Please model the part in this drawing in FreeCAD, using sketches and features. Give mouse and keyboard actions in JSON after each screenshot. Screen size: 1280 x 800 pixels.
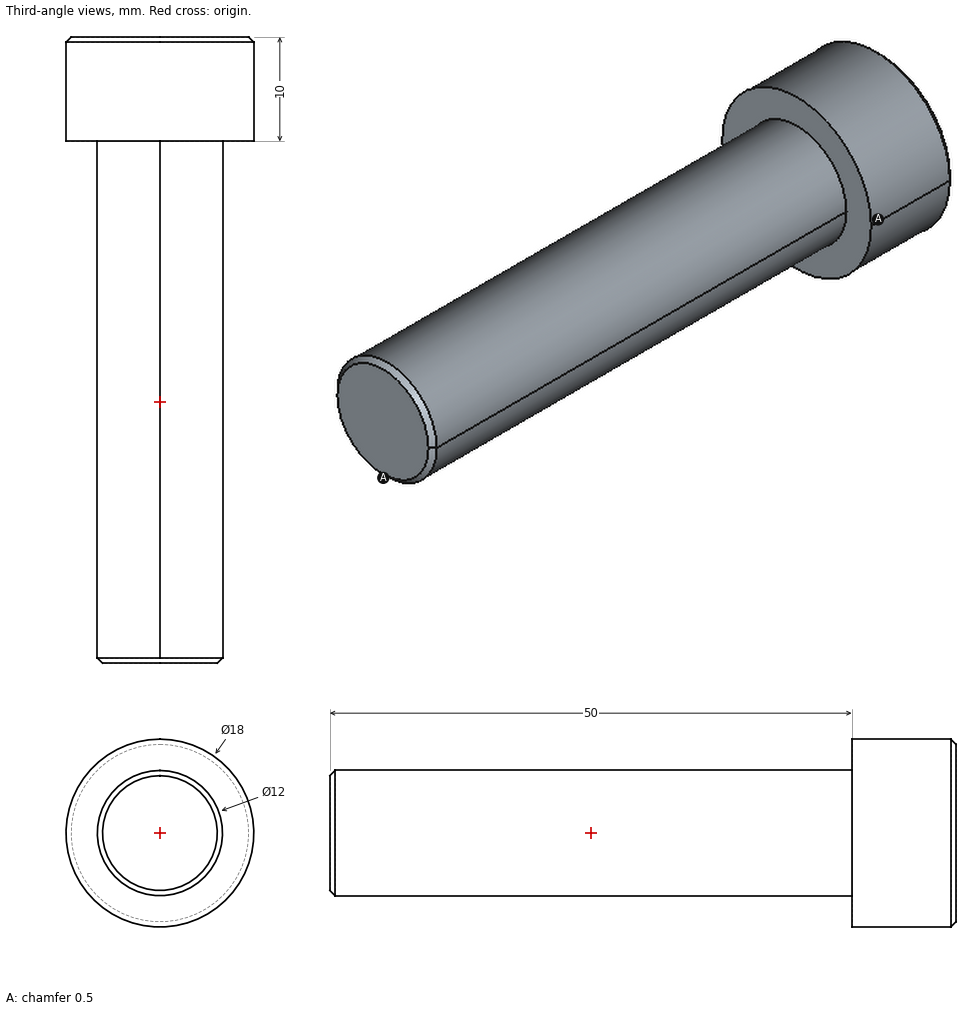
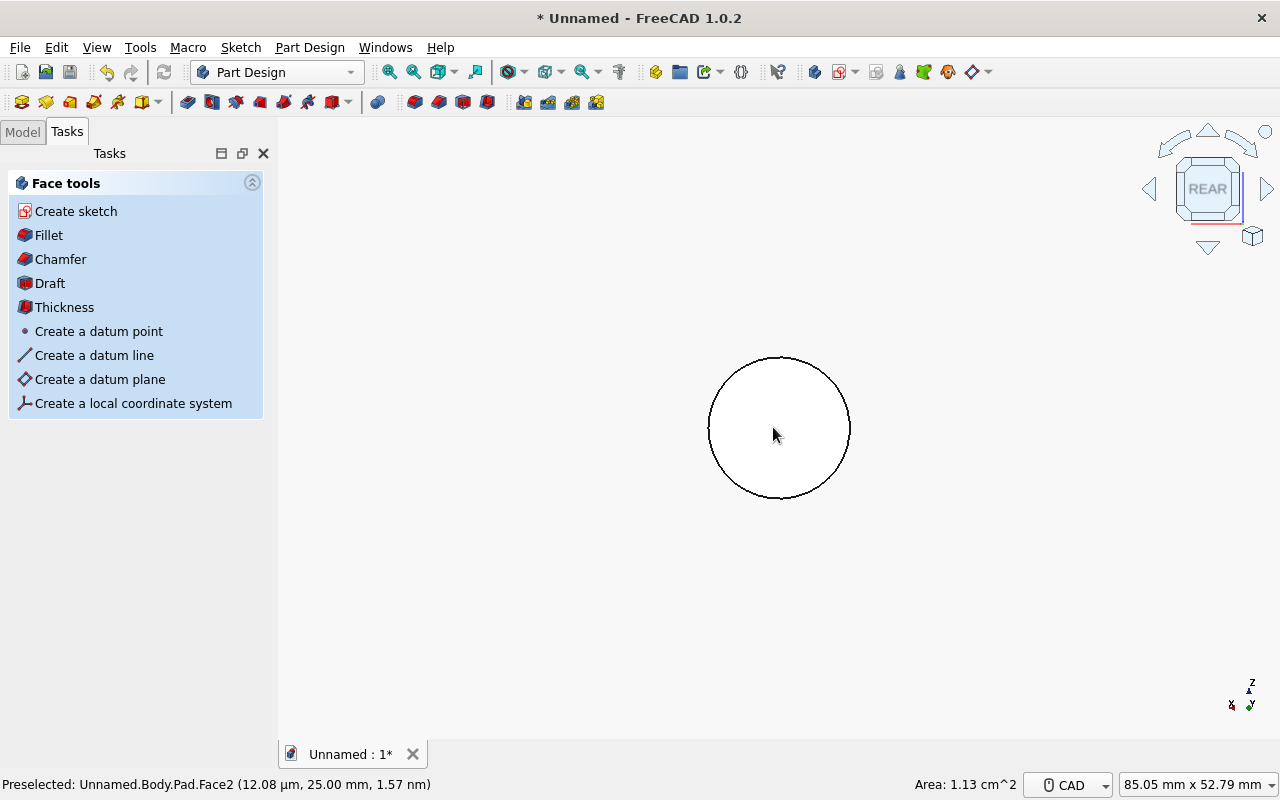
{"action": "left_click", "coordinate": [840, 72]}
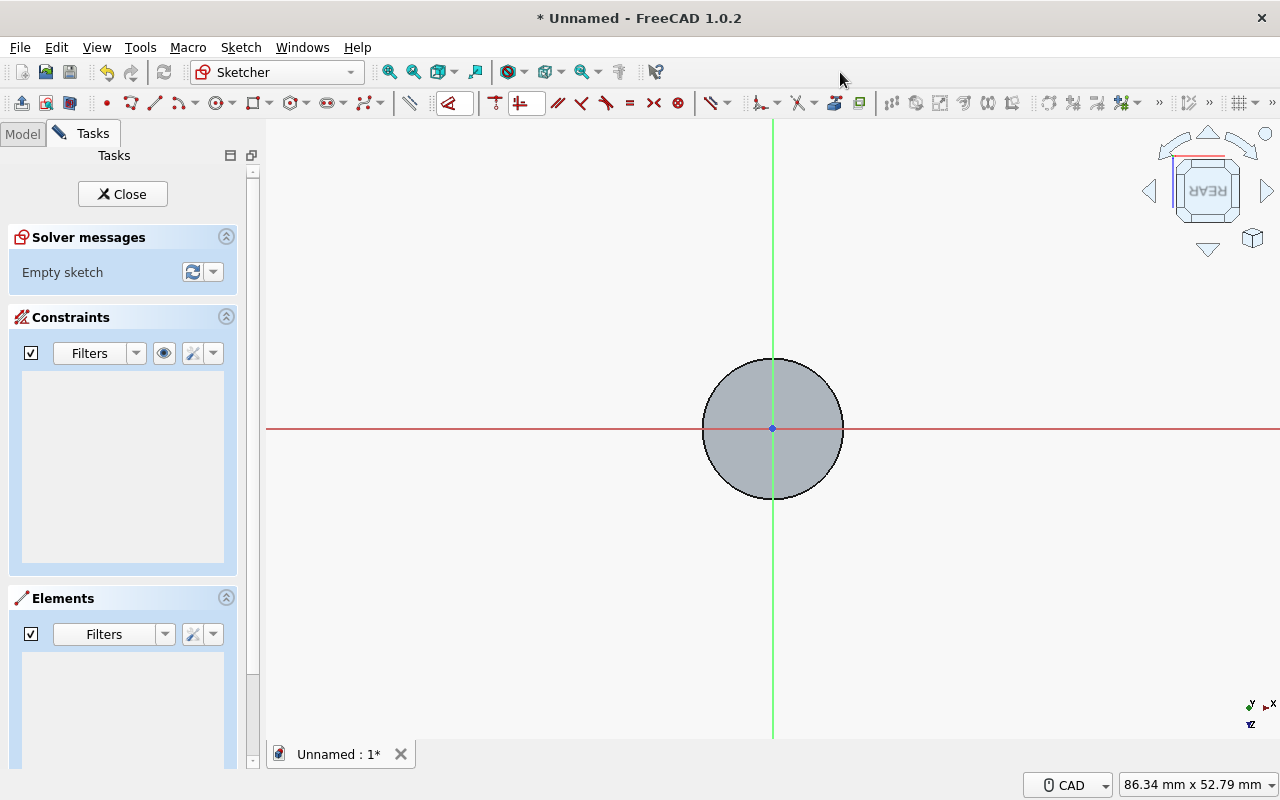
{"action": "scroll", "coordinate": [856, 429], "scroll_direction": "up", "scroll_amount": 3}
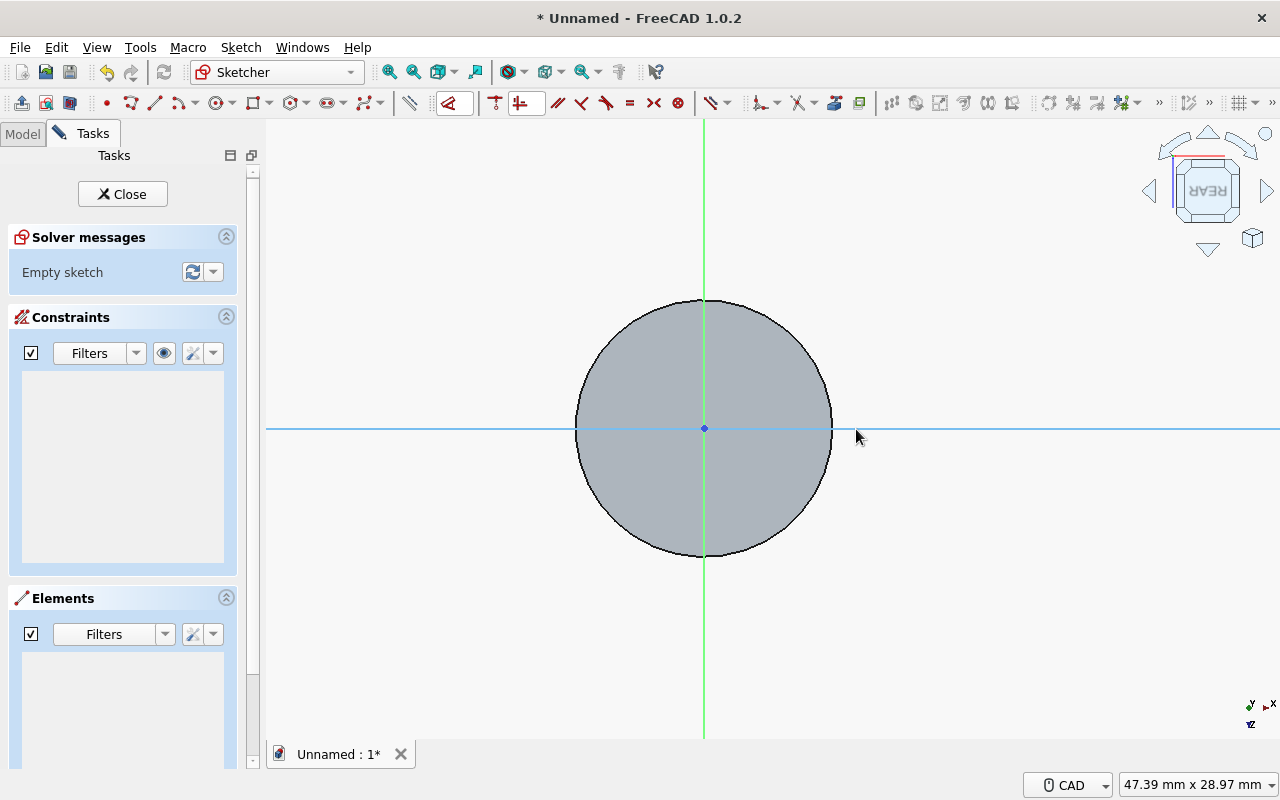
{"action": "left_click", "coordinate": [216, 104]}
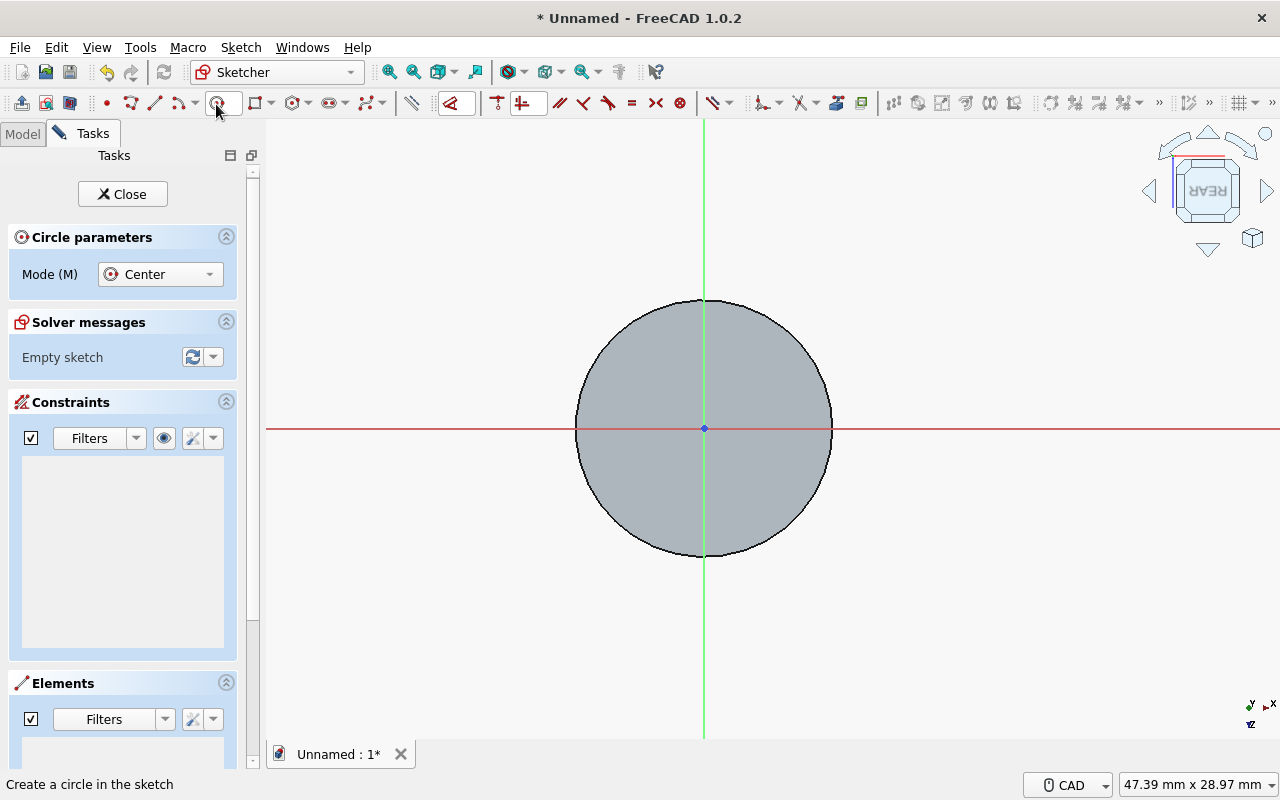
{"action": "left_click", "coordinate": [704, 429]}
{"action": "left_click", "coordinate": [840, 292]}
{"action": "key", "text": "Escape"}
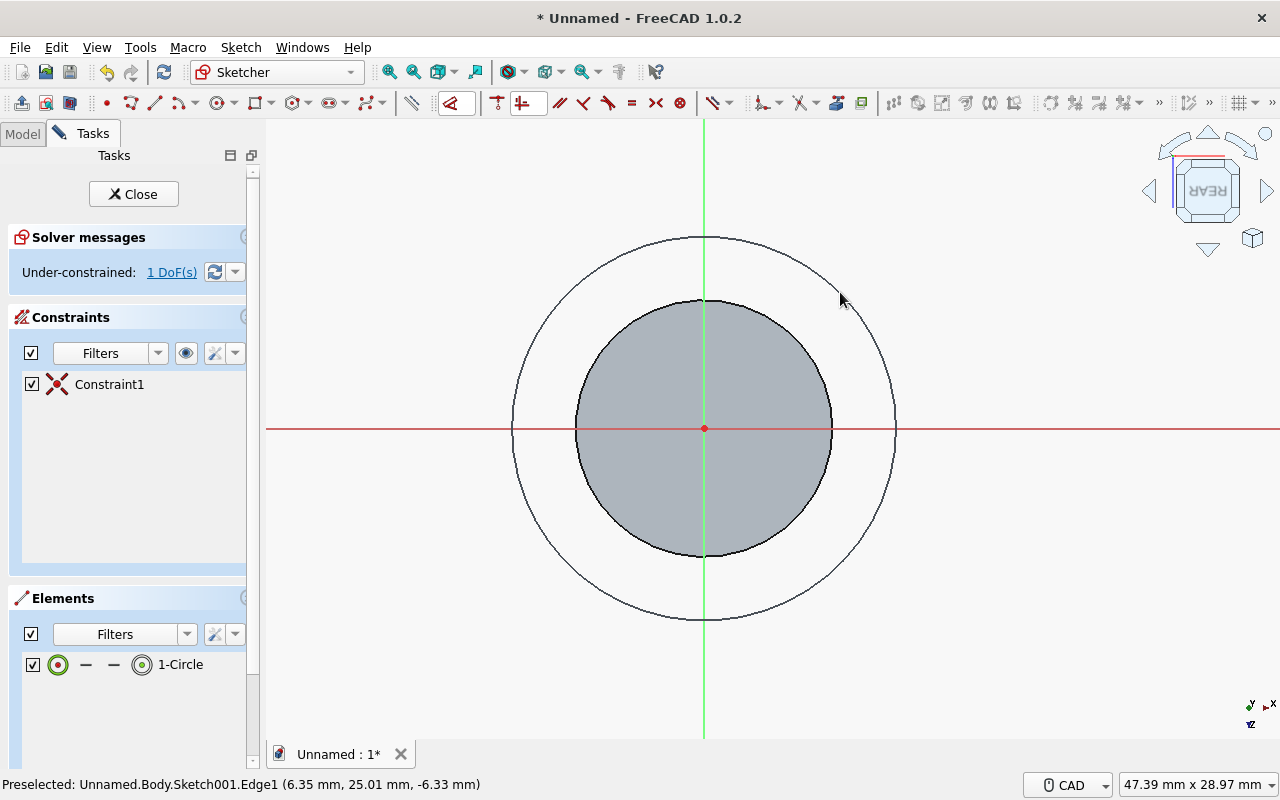
{"action": "left_click", "coordinate": [839, 292]}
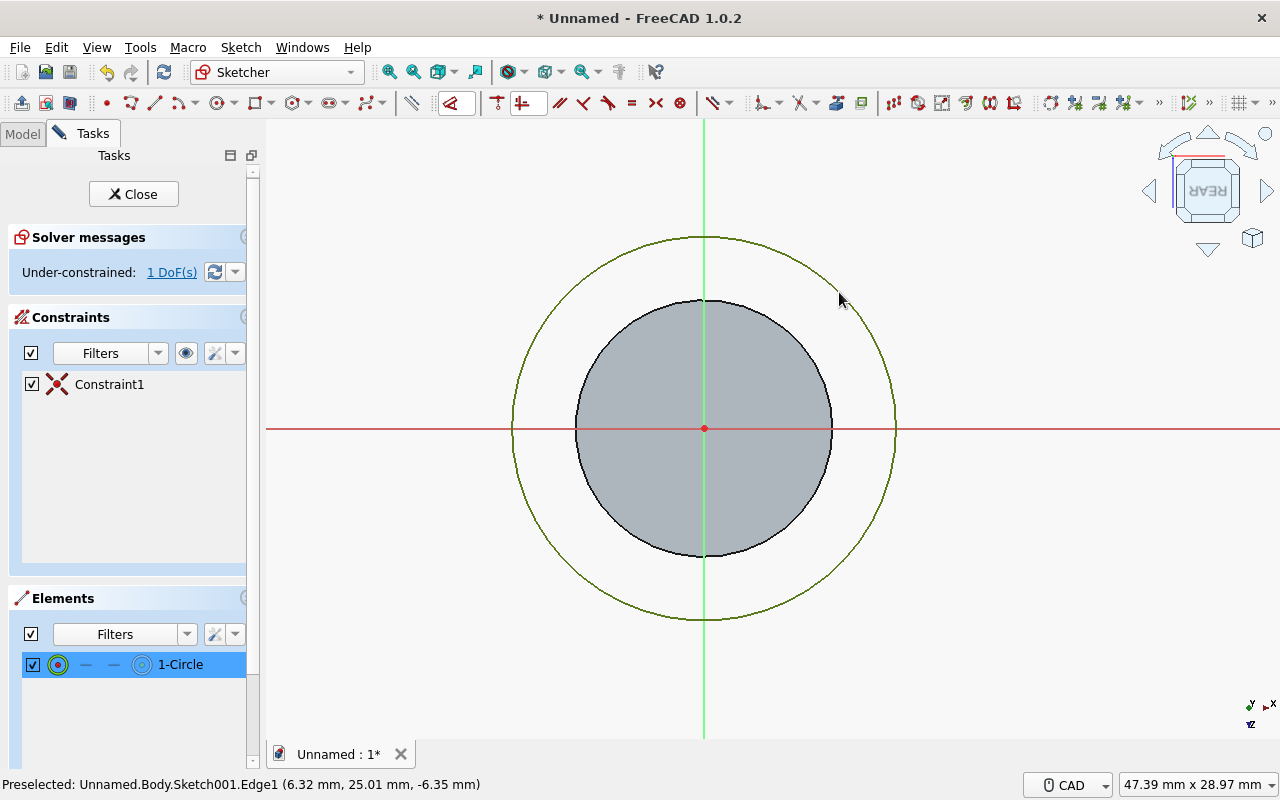
{"action": "left_click", "coordinate": [470, 104]}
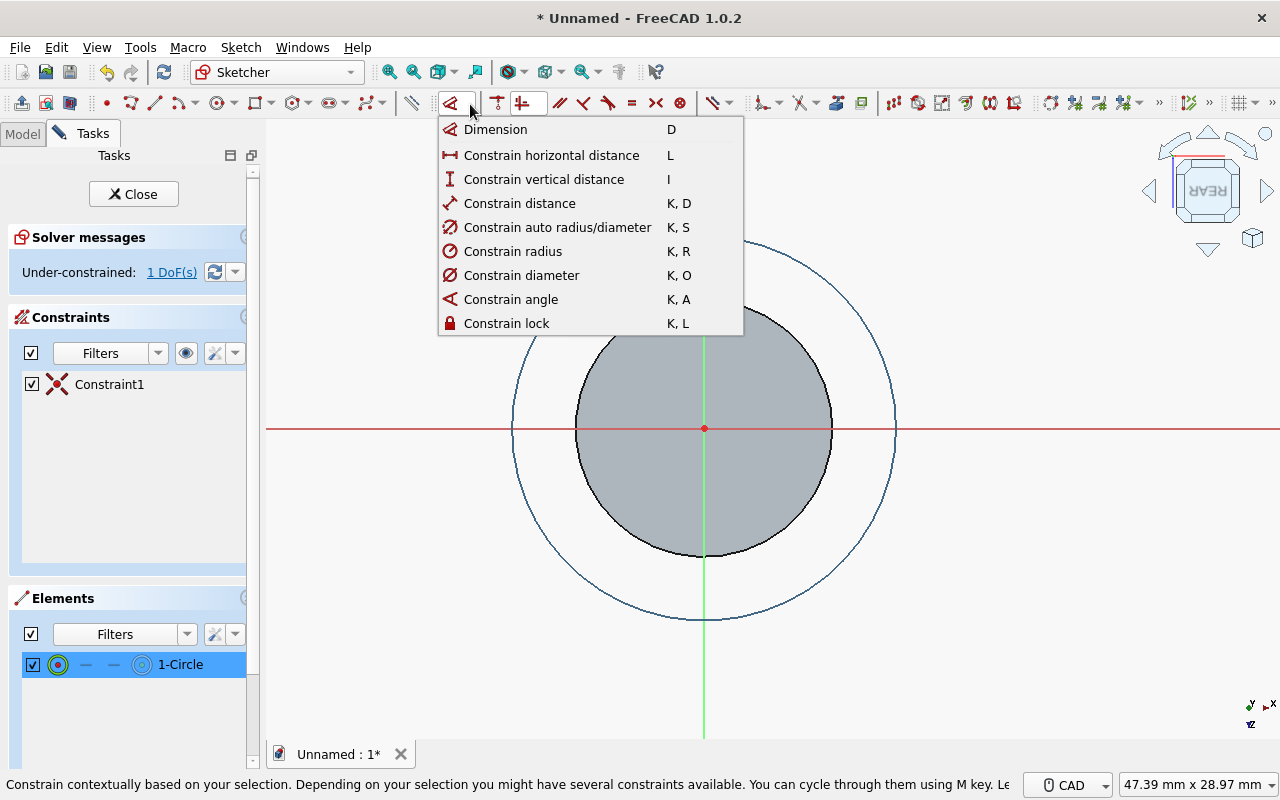
{"action": "left_click", "coordinate": [591, 275]}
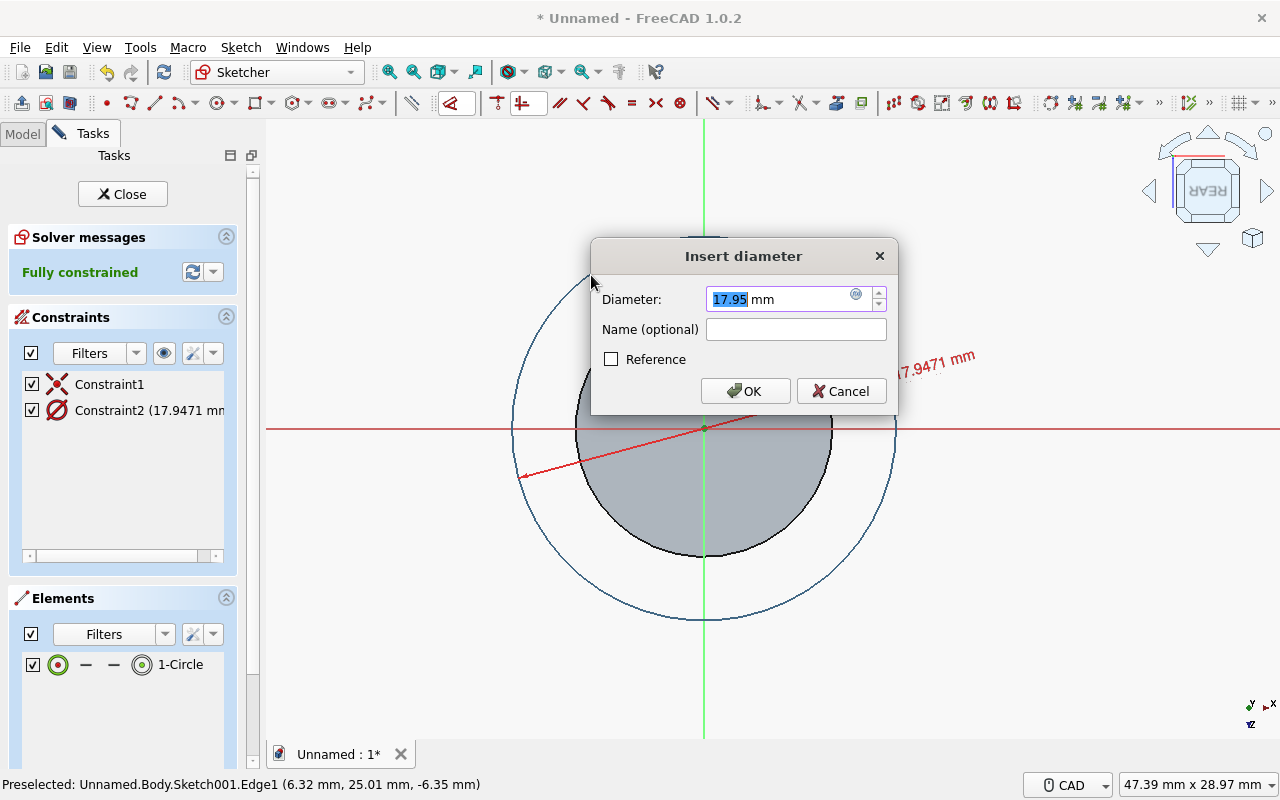
{"action": "type", "text": "18"}
{"action": "key", "text": "Return"}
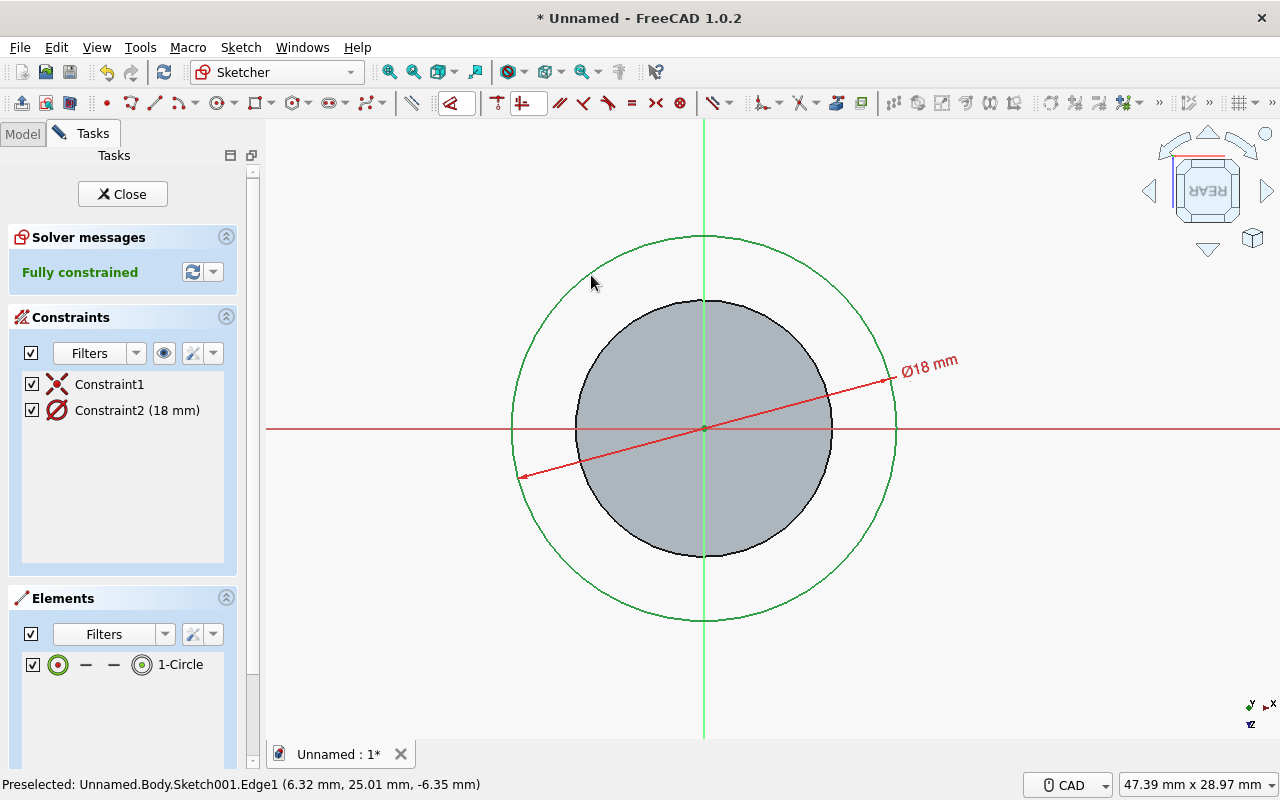
{"action": "left_click", "coordinate": [123, 194]}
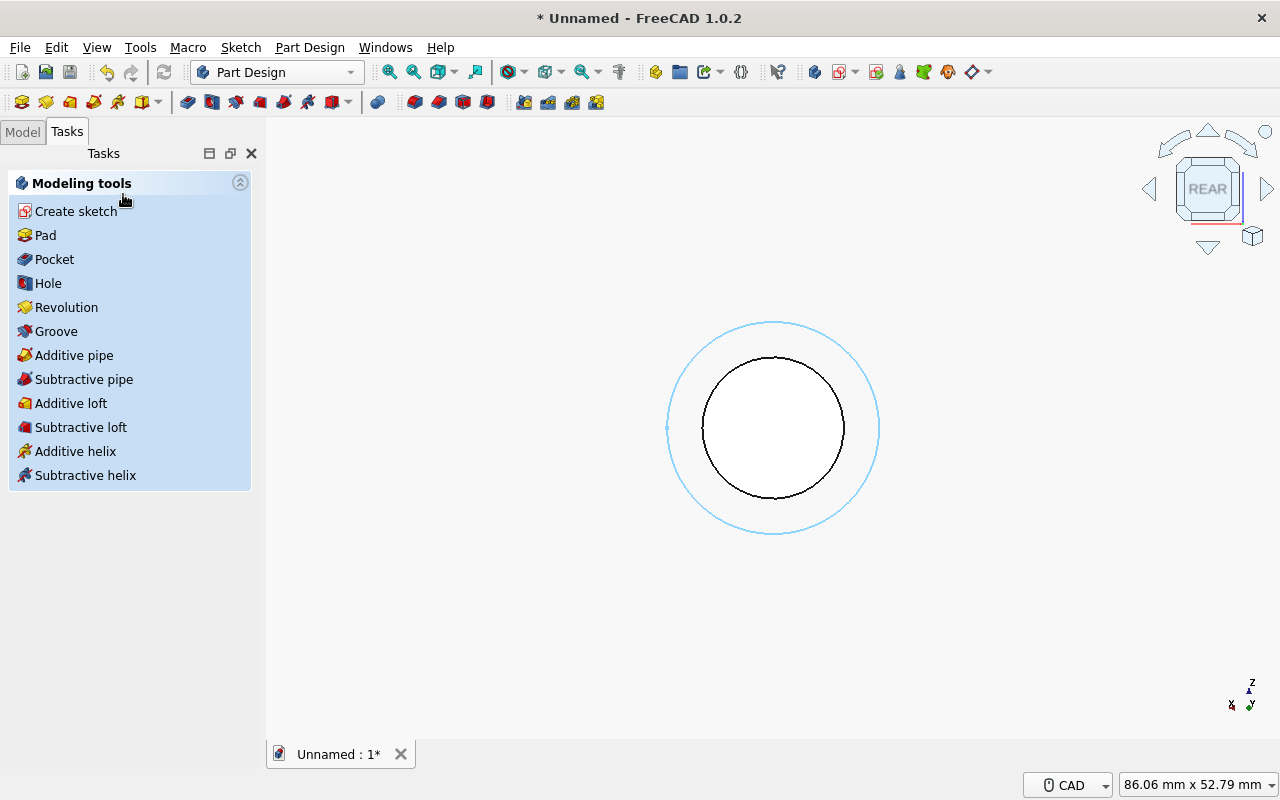
{"action": "left_click", "coordinate": [22, 102]}